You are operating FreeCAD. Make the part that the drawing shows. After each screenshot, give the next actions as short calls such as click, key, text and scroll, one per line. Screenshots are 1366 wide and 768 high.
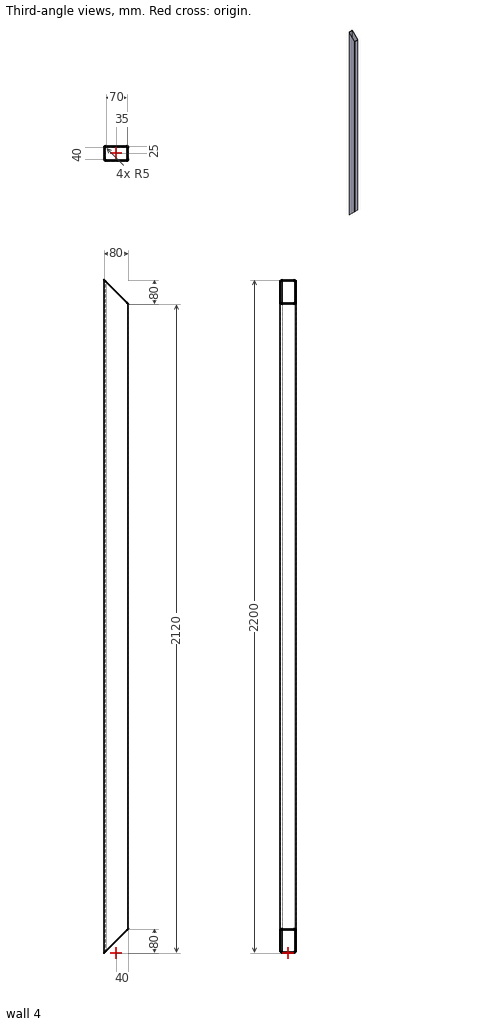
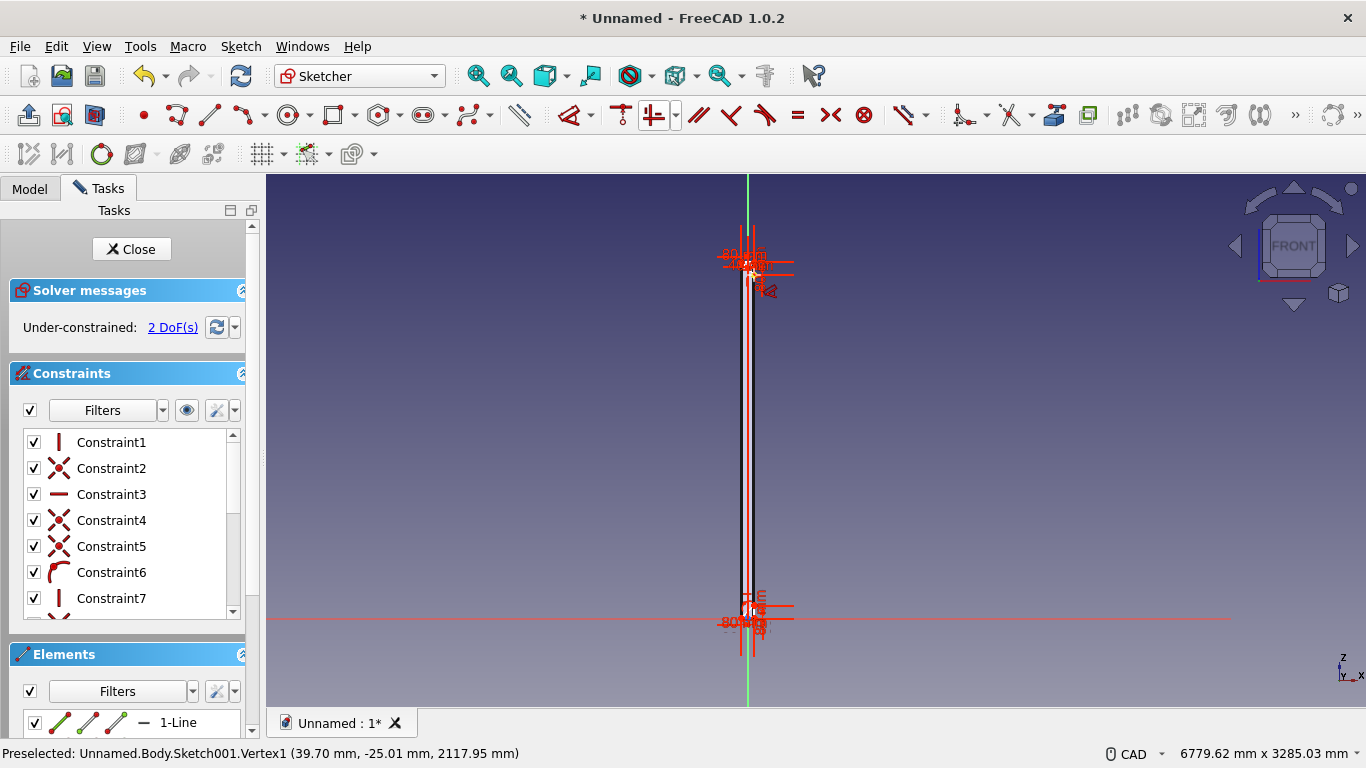
scroll(754, 619, up, 10)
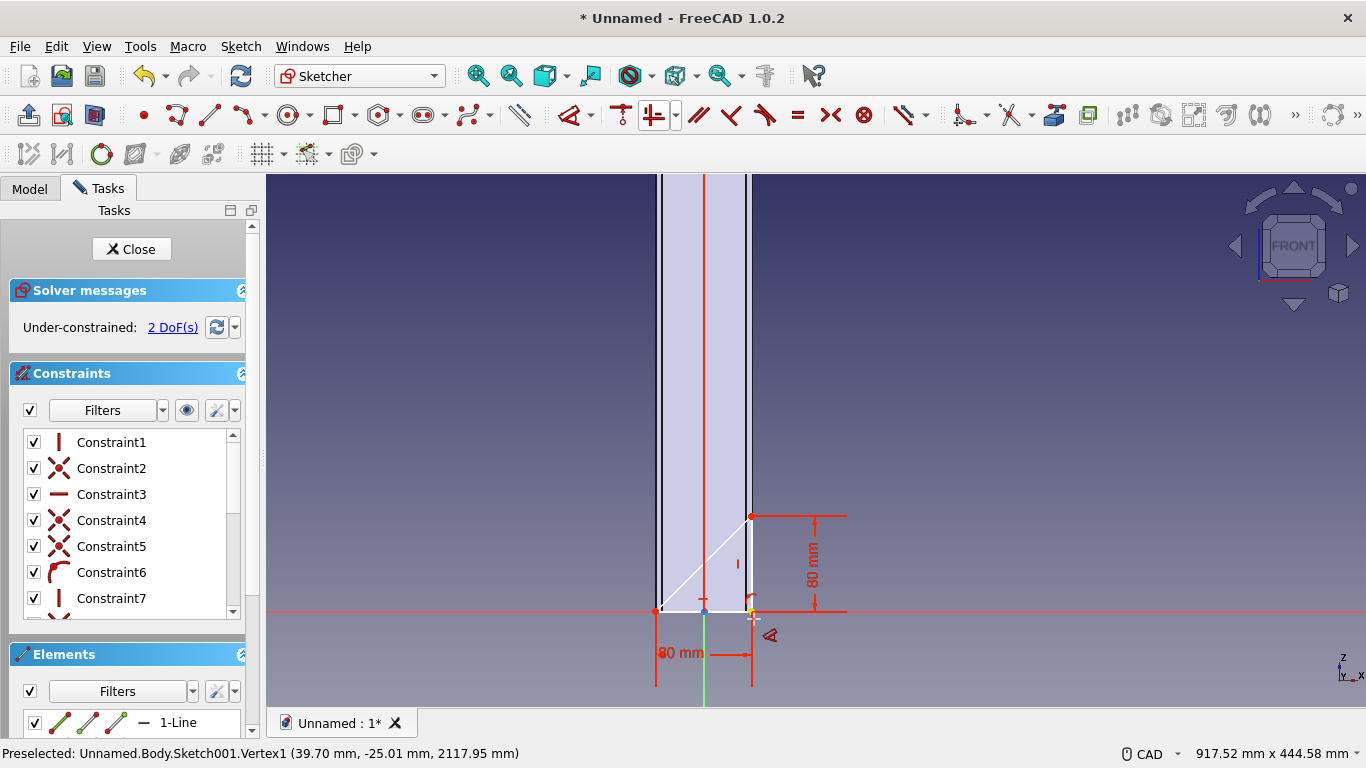
click(752, 612)
click(728, 578)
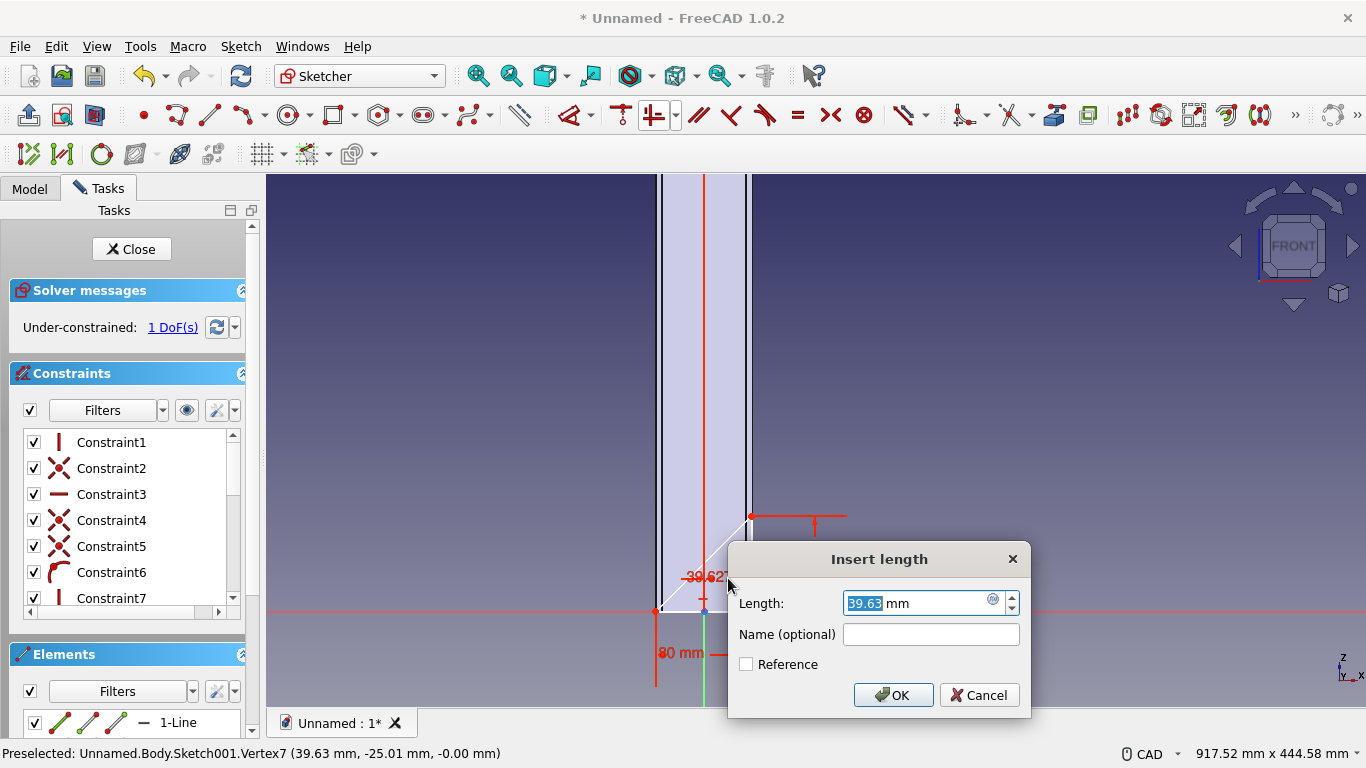
text(40)
key(Return)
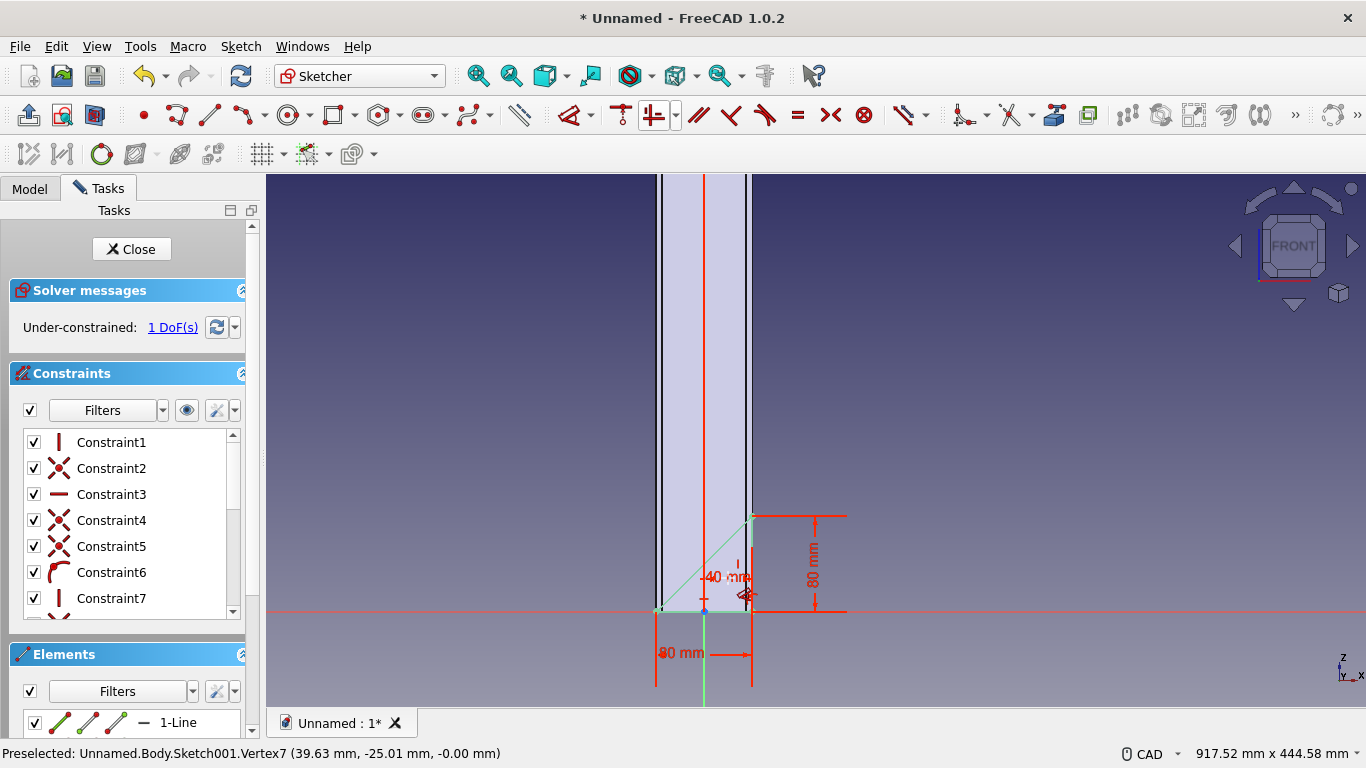
scroll(754, 620, down, 10)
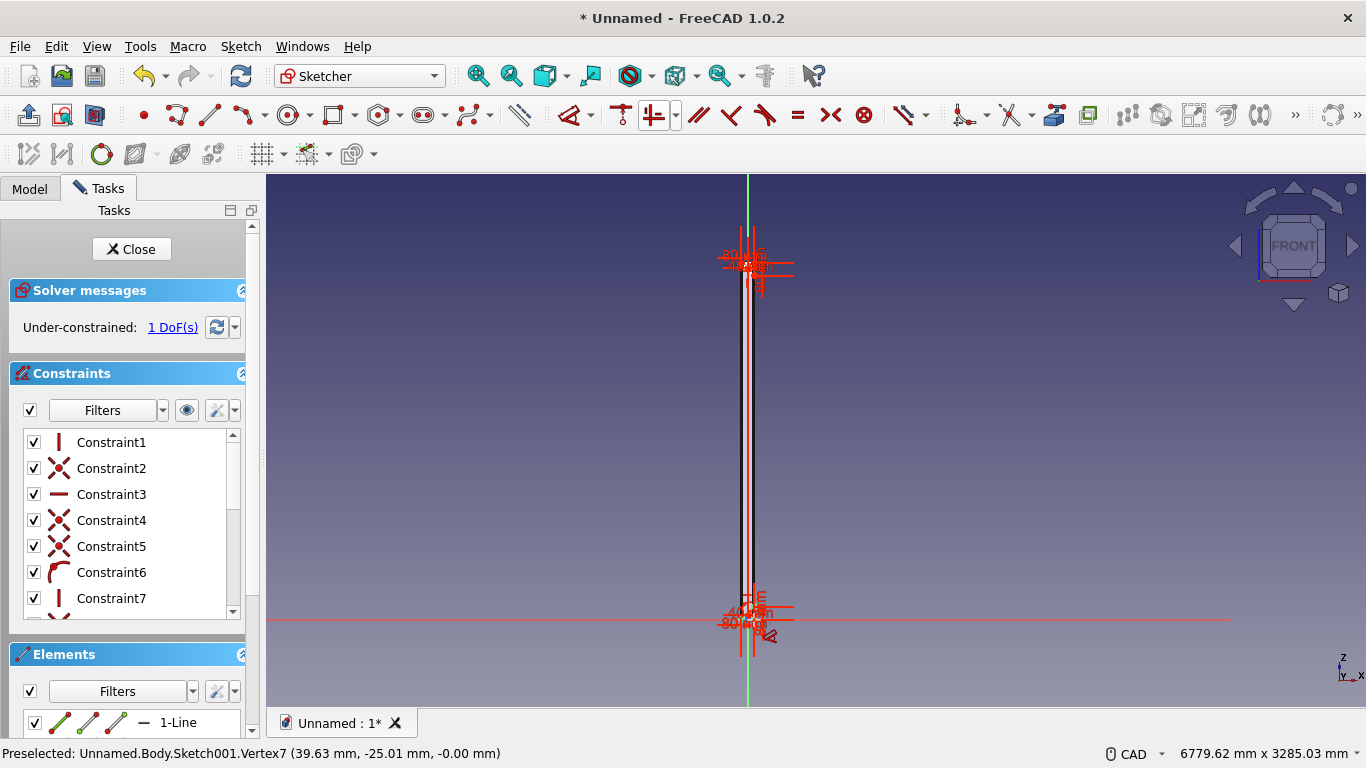
click(754, 276)
click(788, 448)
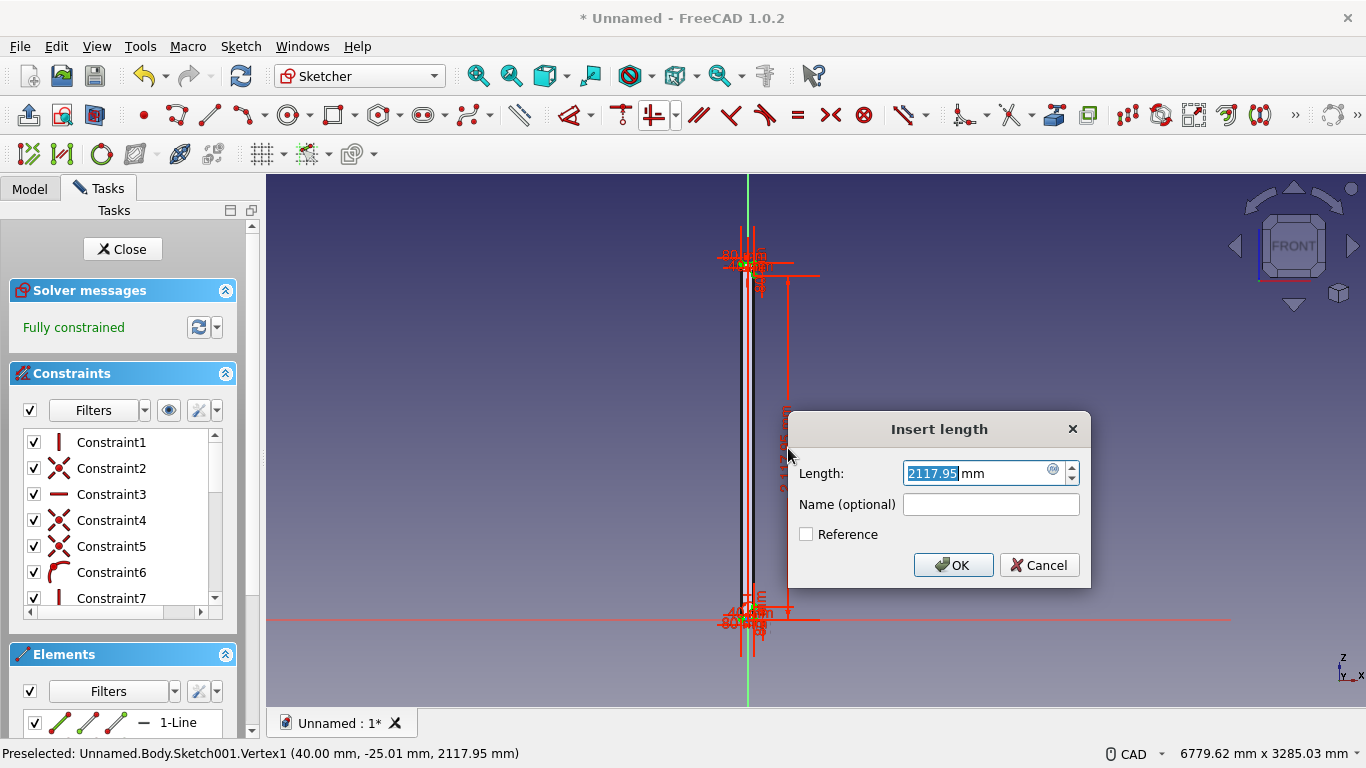
text(2120)
key(Return)
key(Escape)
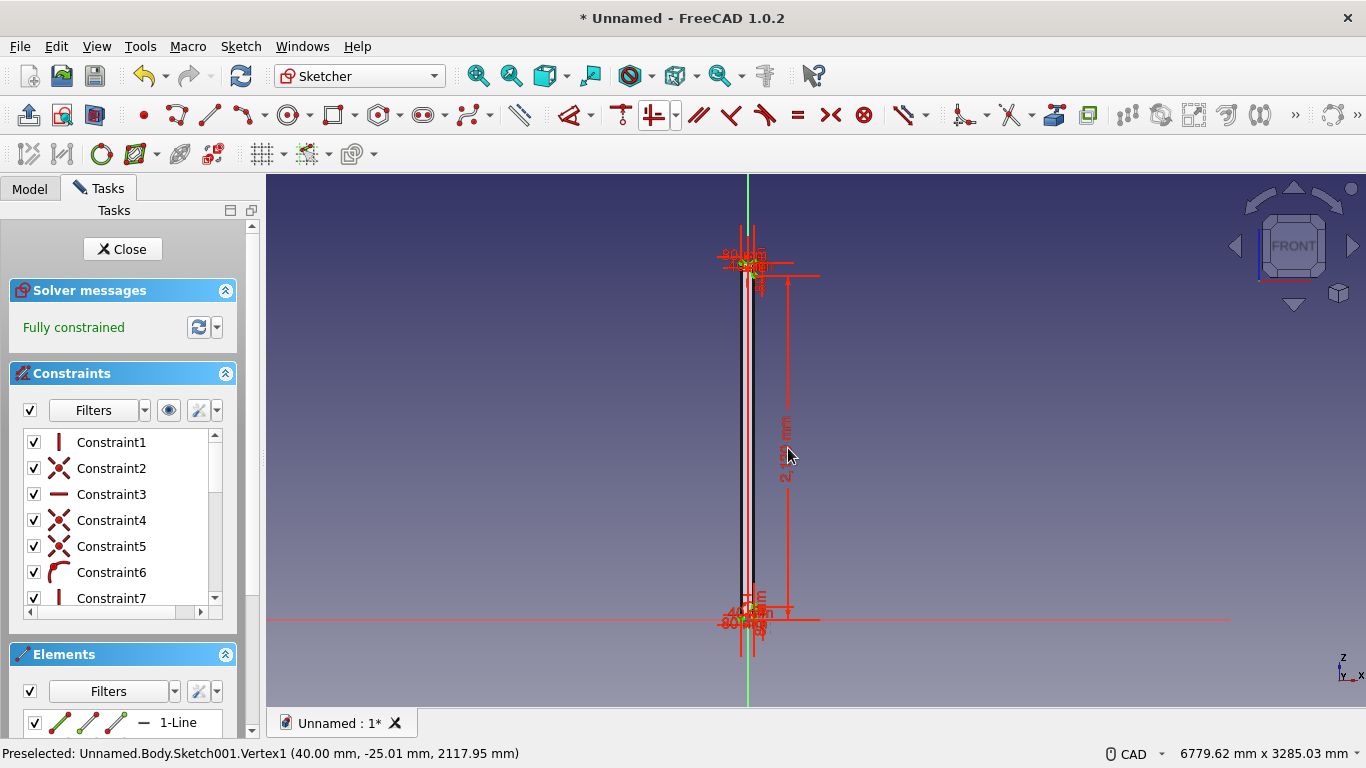
click(123, 249)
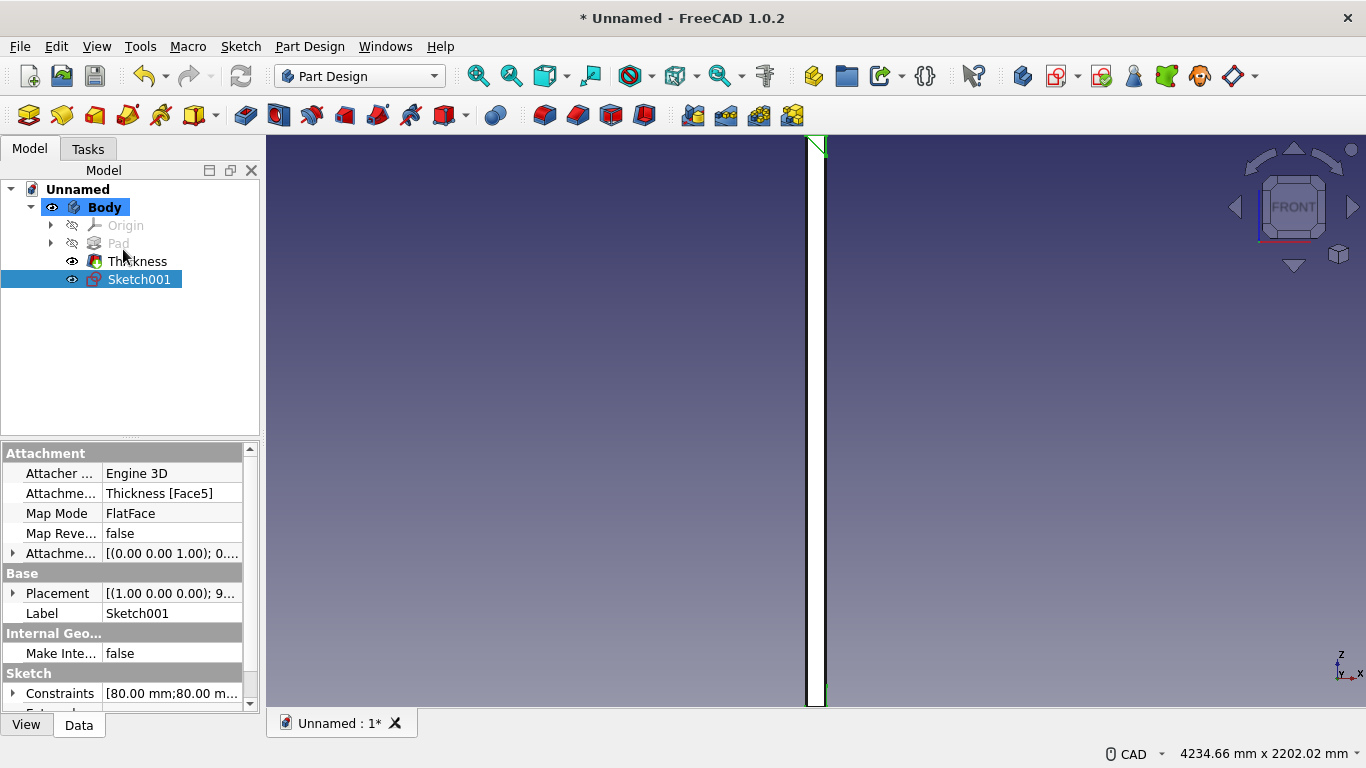
click(246, 116)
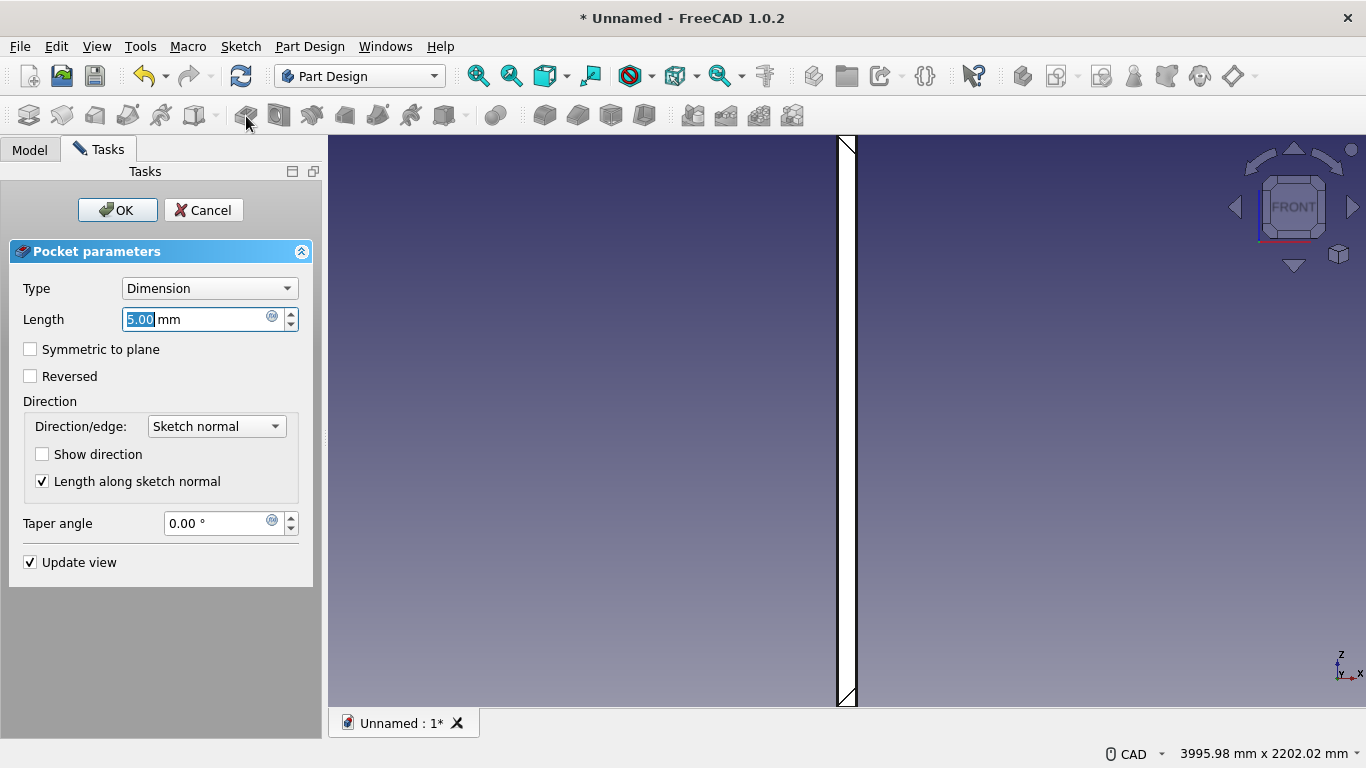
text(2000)
key(Tab)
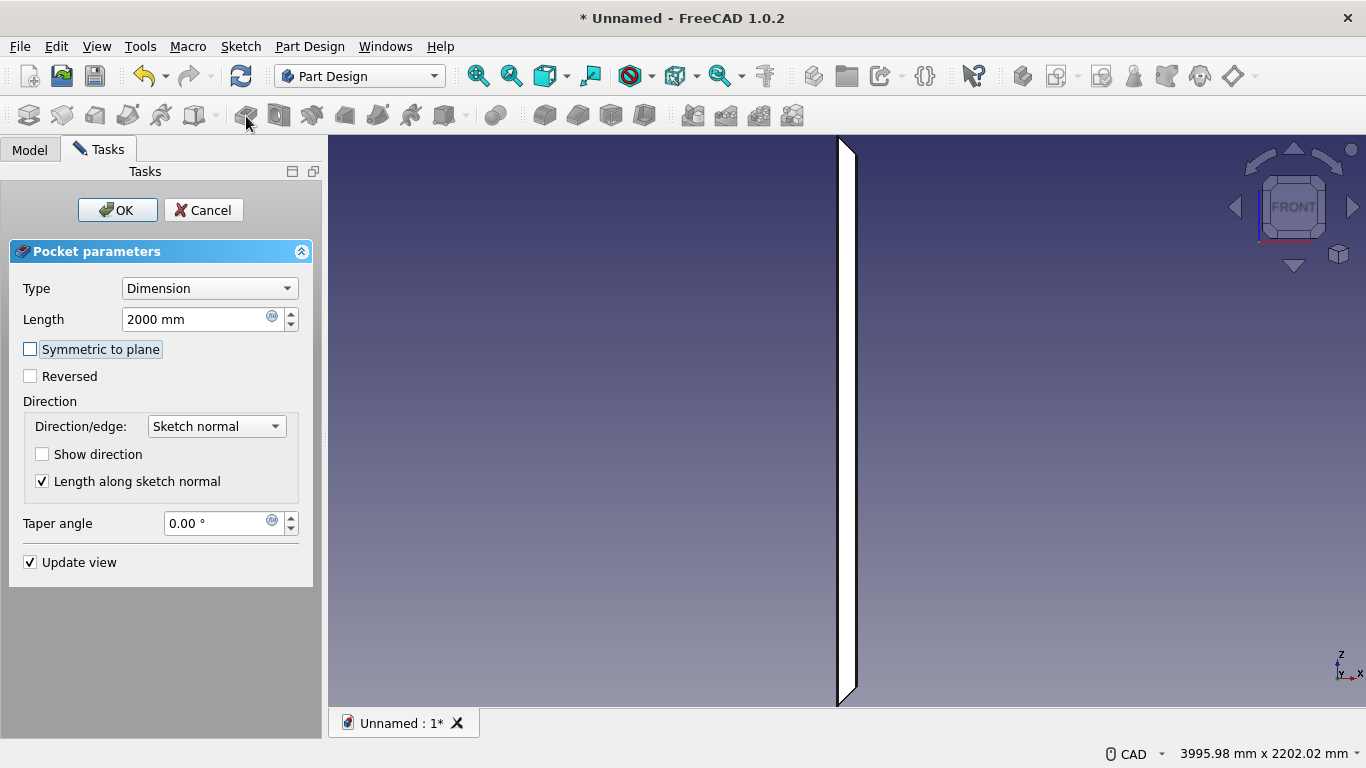
click(118, 210)